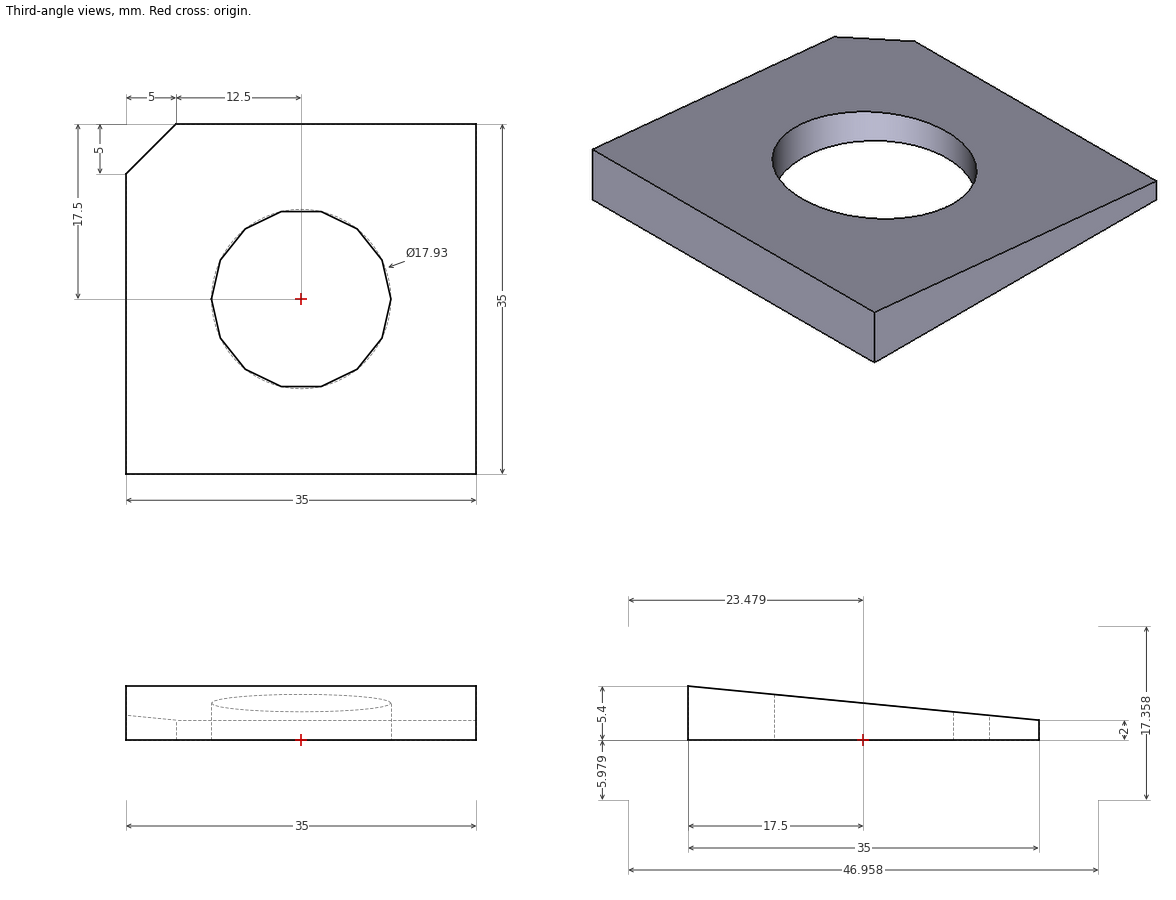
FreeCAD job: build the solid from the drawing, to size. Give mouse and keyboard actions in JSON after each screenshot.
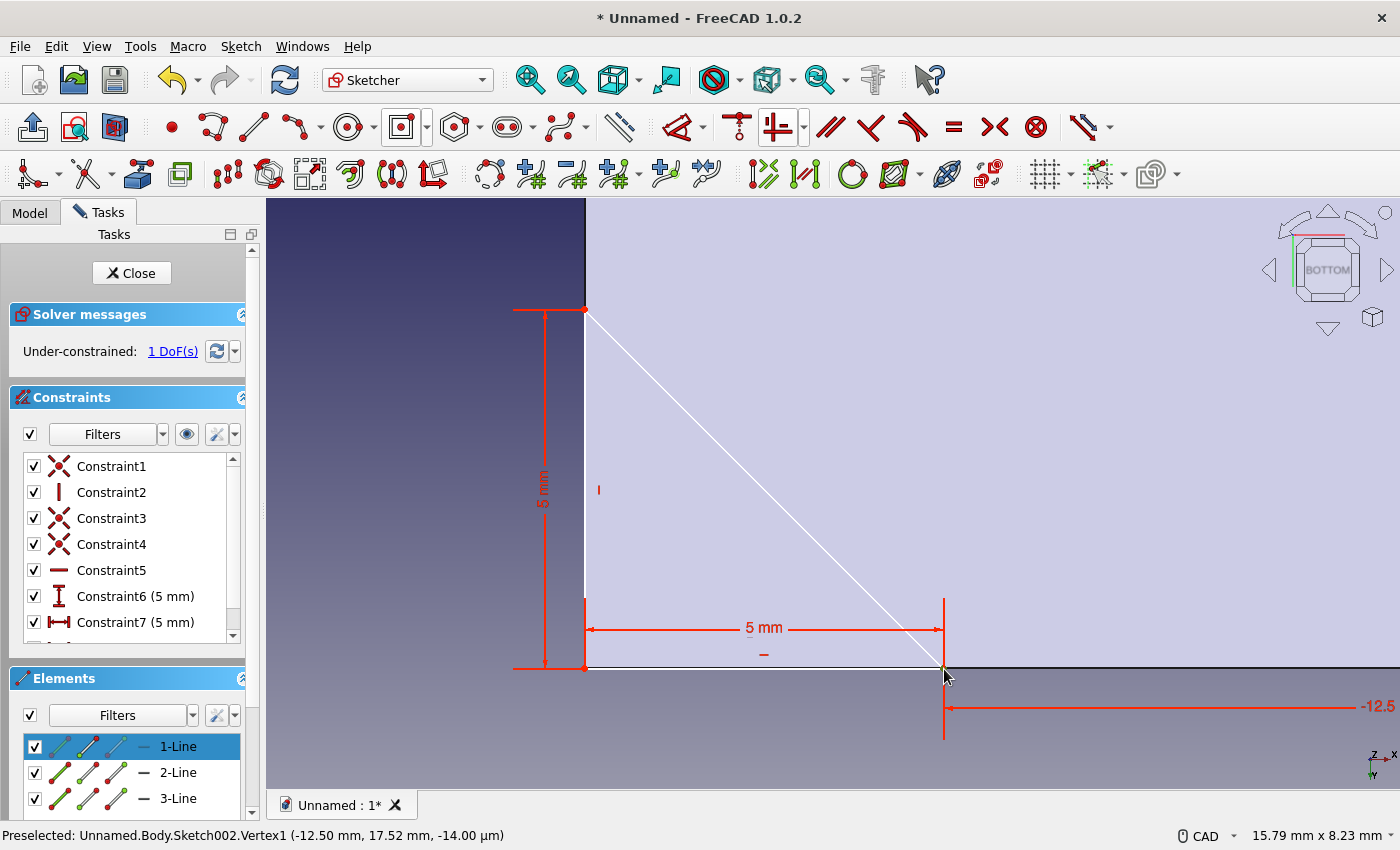
{"action": "key", "text": "i"}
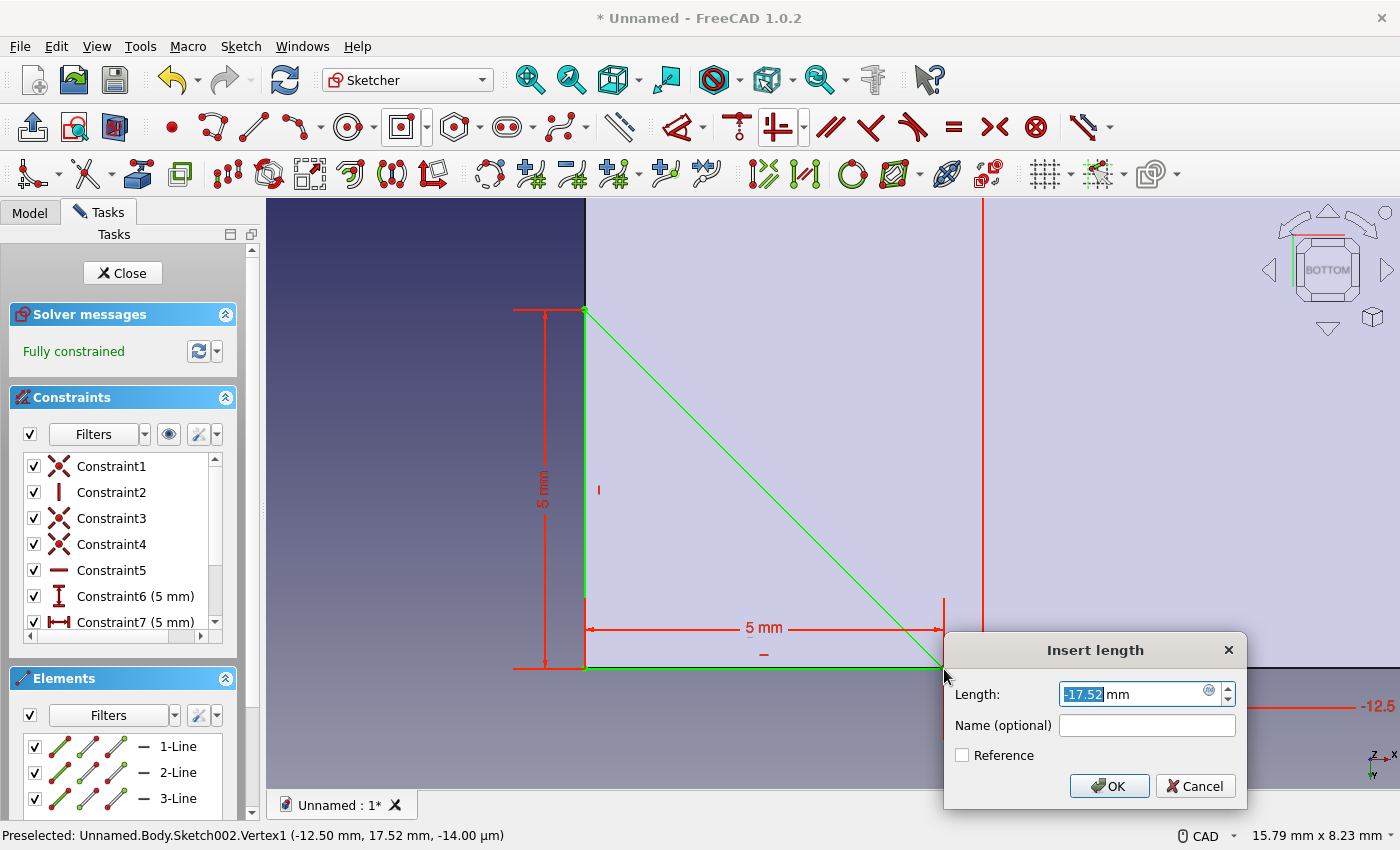
{"action": "type", "text": "-17.5"}
{"action": "key", "text": "Return"}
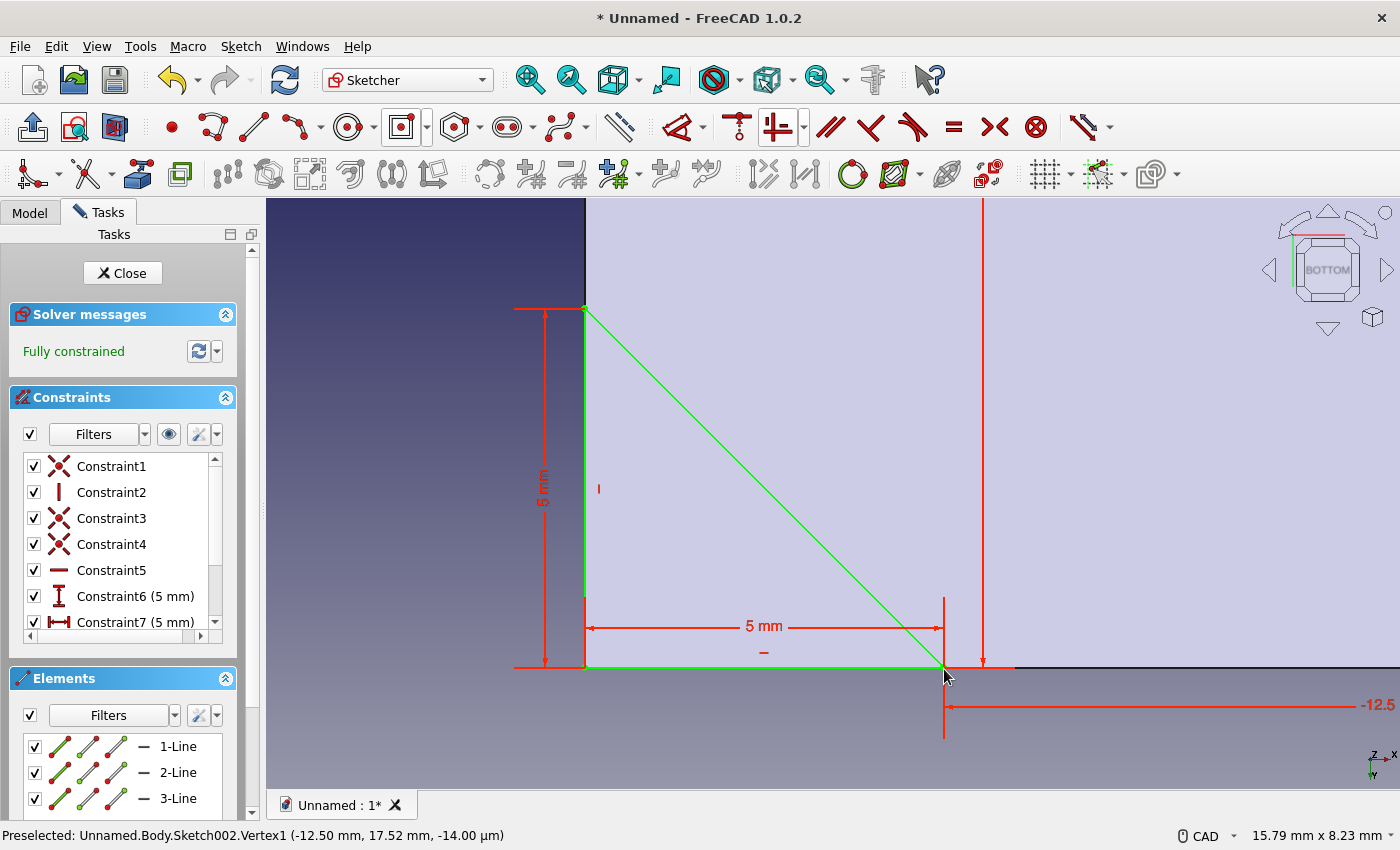
{"action": "left_click", "coordinate": [123, 273]}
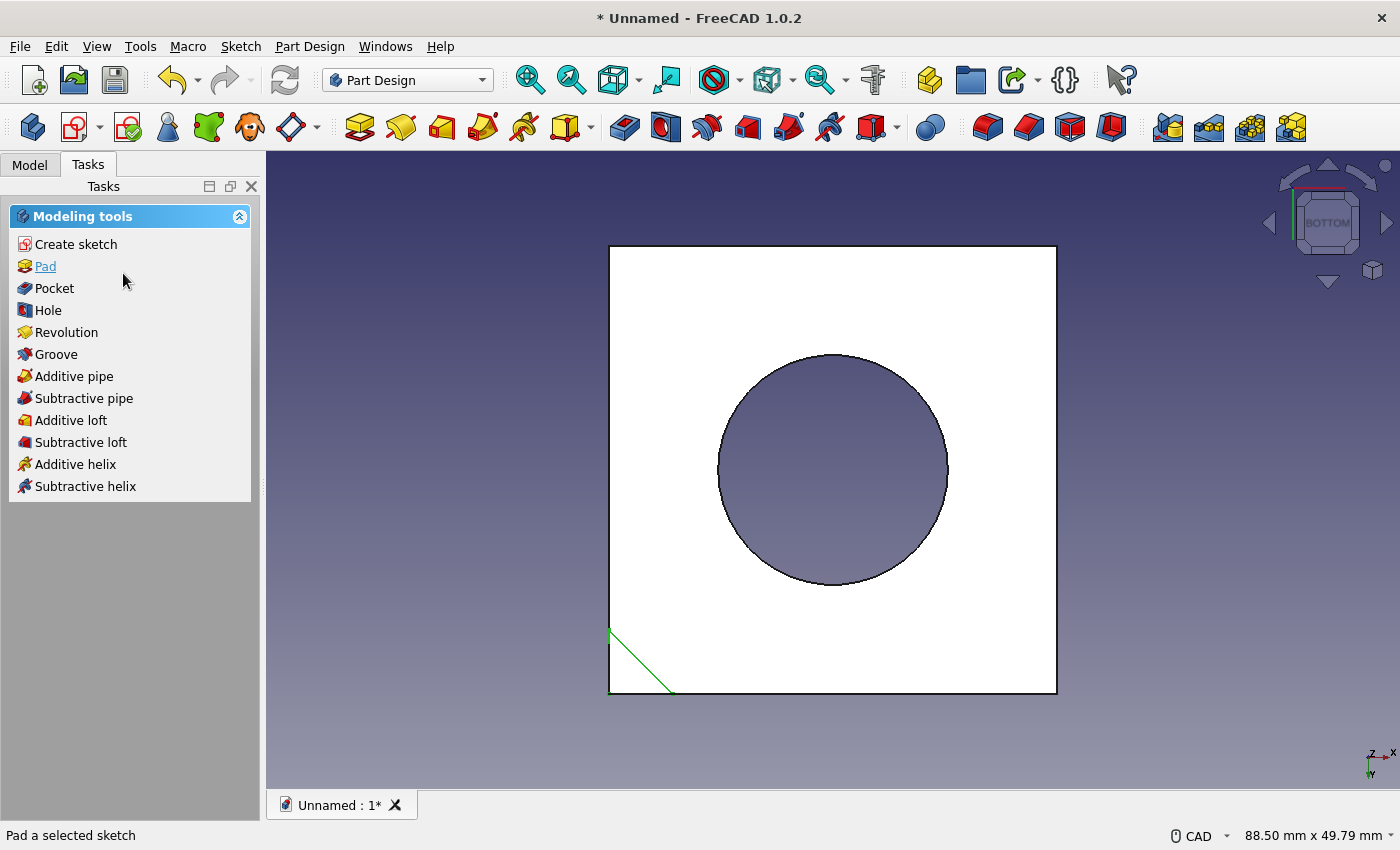
{"action": "left_click", "coordinate": [625, 128]}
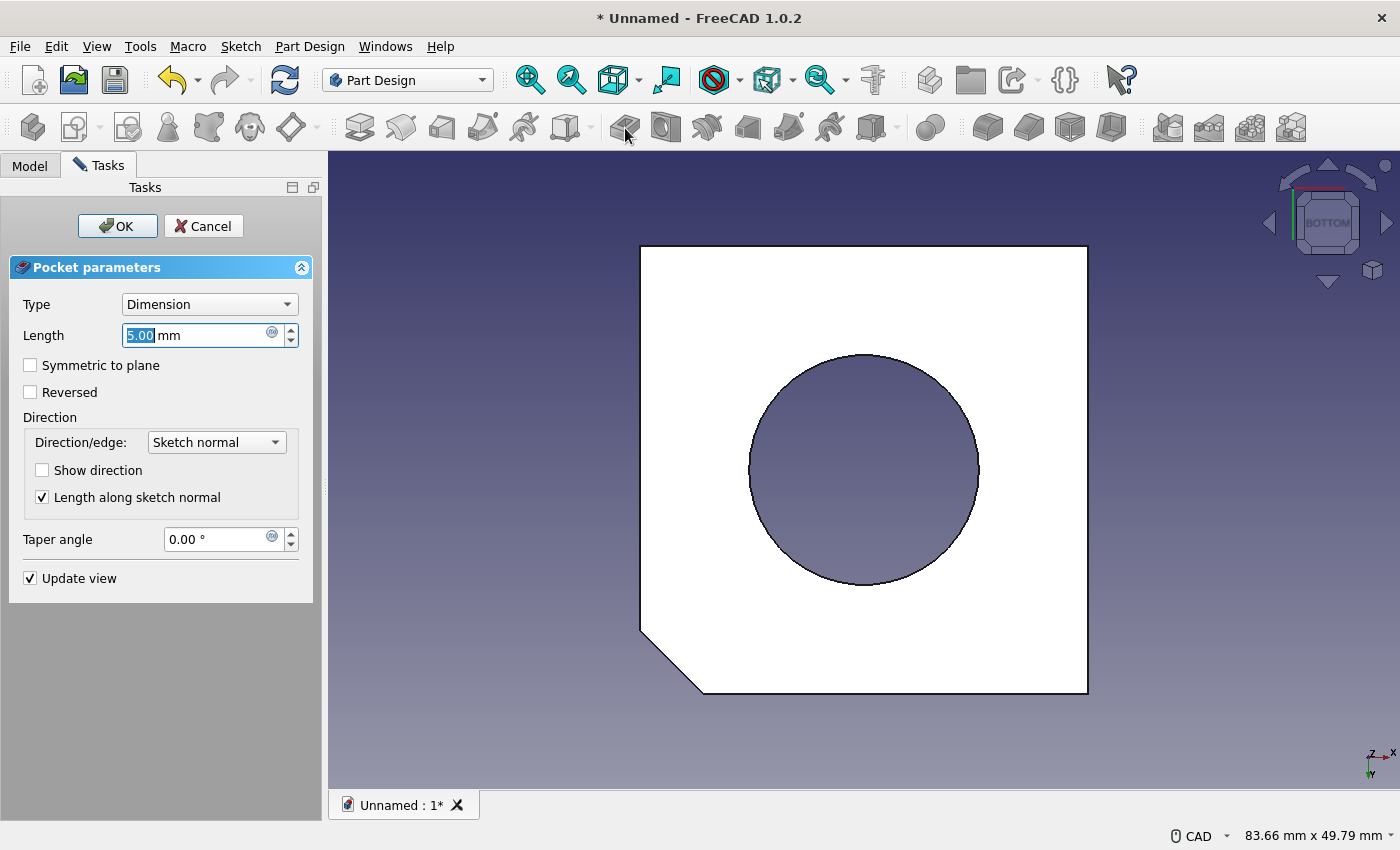
{"action": "left_click", "coordinate": [210, 304]}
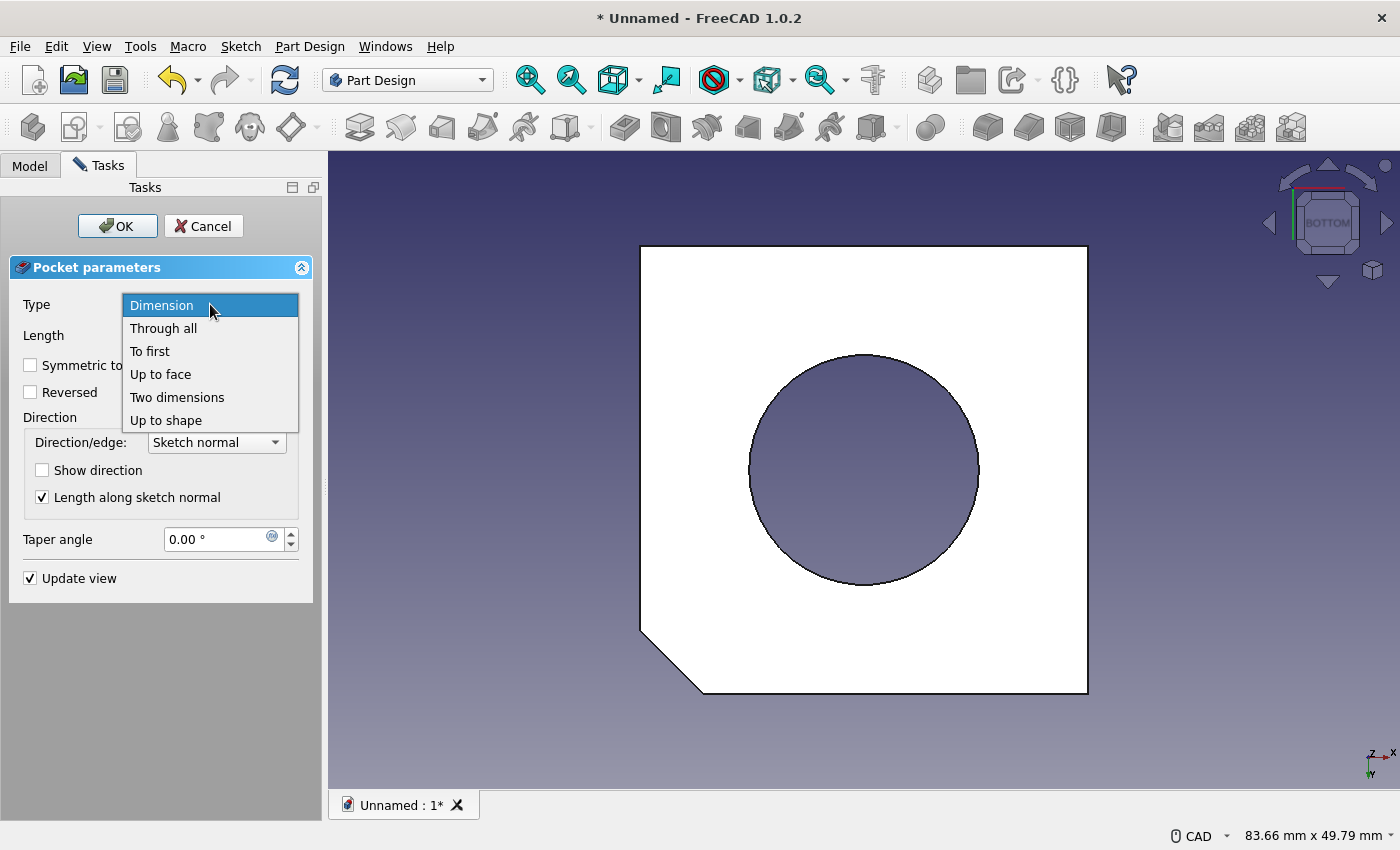
{"action": "left_click", "coordinate": [208, 328]}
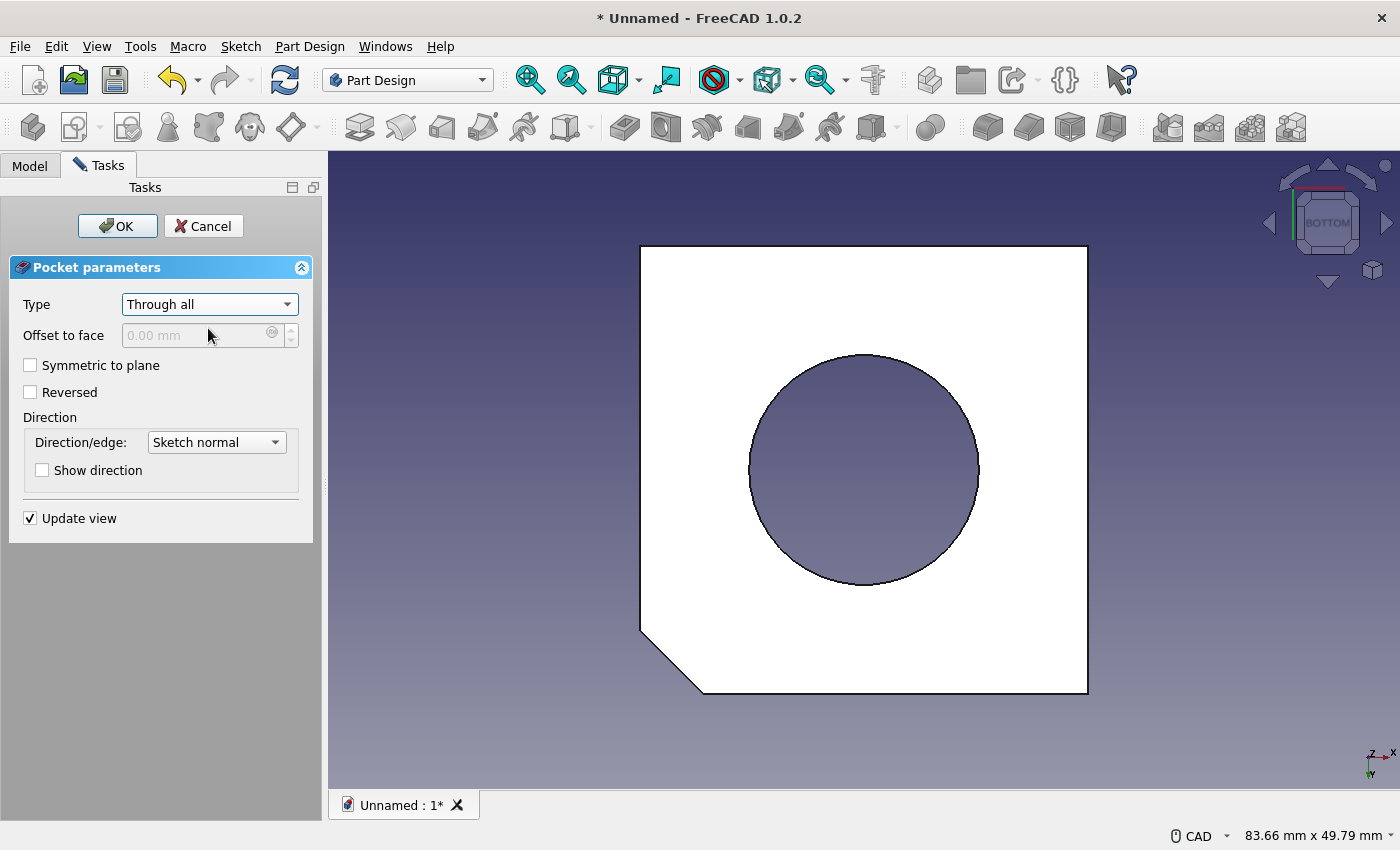
{"action": "left_click", "coordinate": [118, 226]}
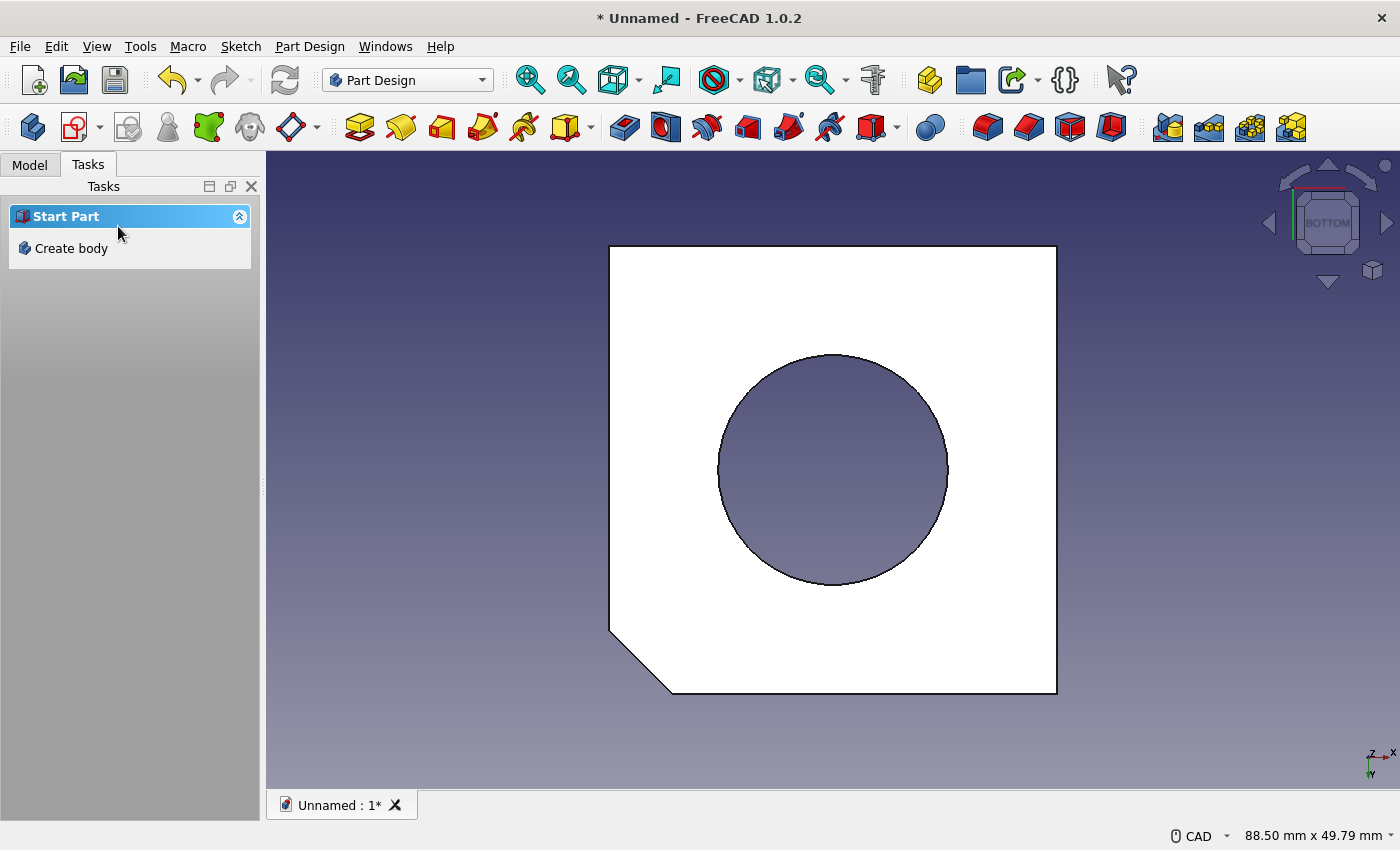
{"action": "key", "text": "0"}